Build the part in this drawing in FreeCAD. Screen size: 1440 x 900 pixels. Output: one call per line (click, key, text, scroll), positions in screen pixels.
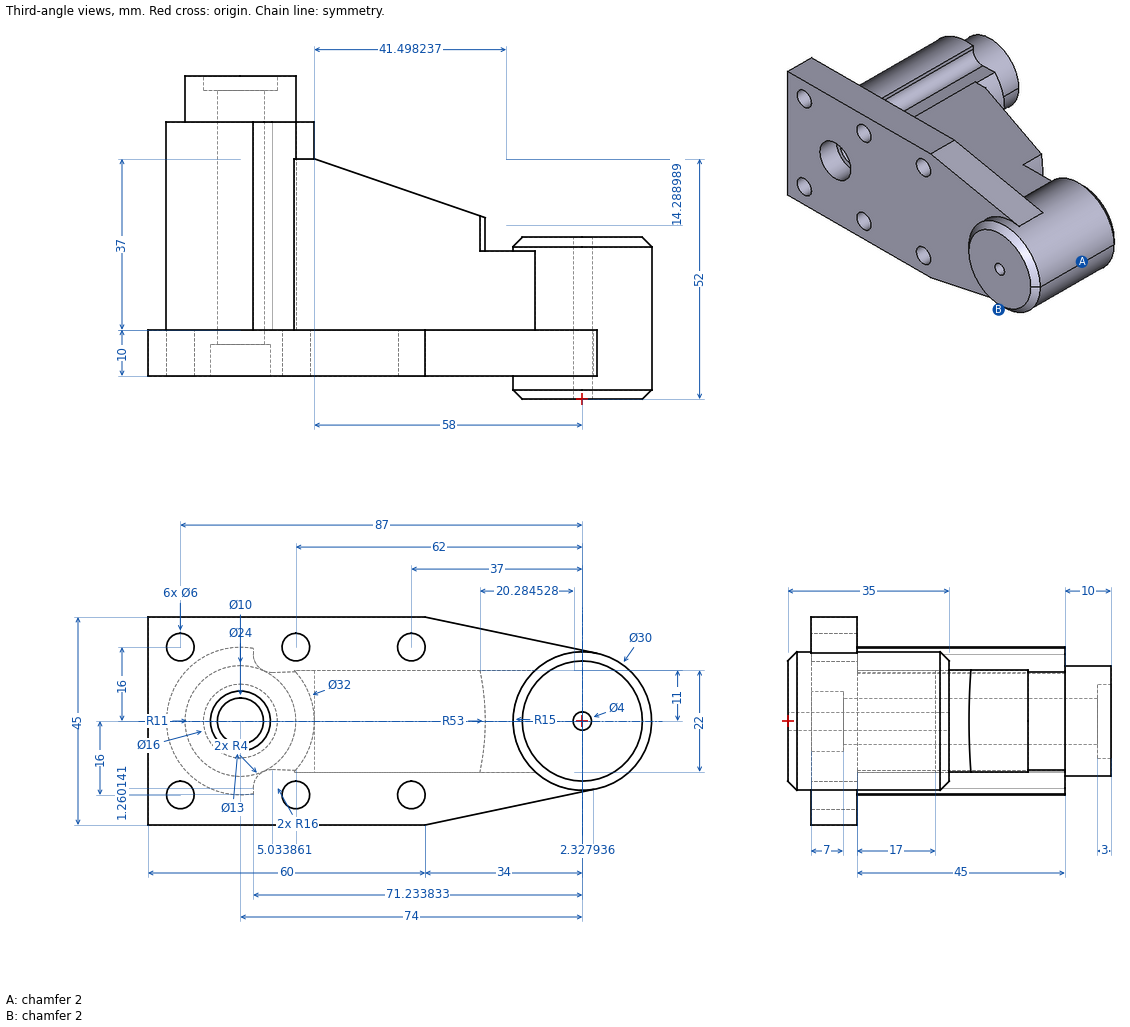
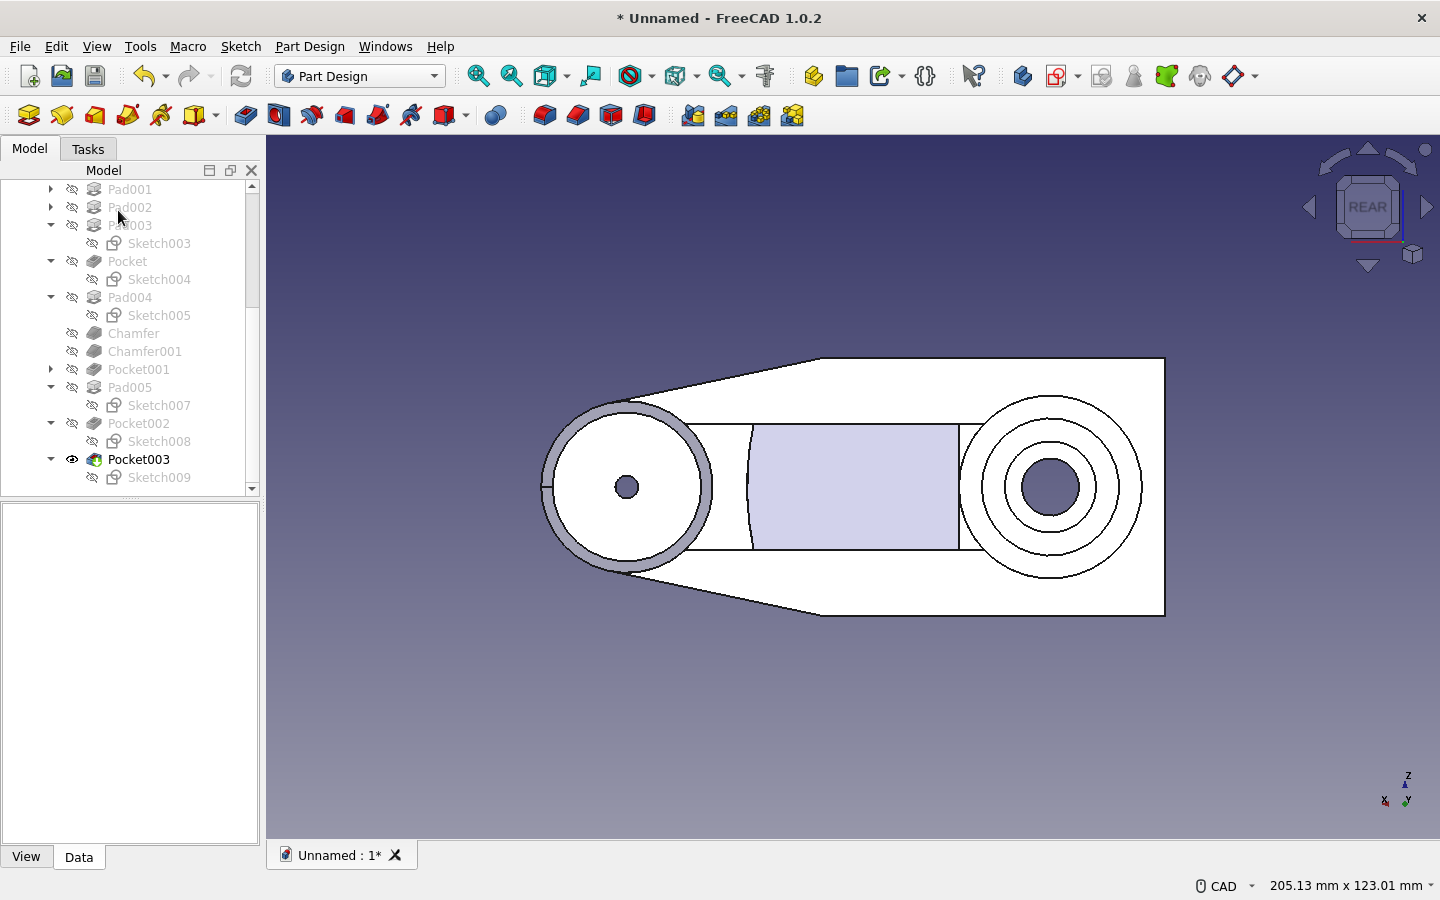
key(0)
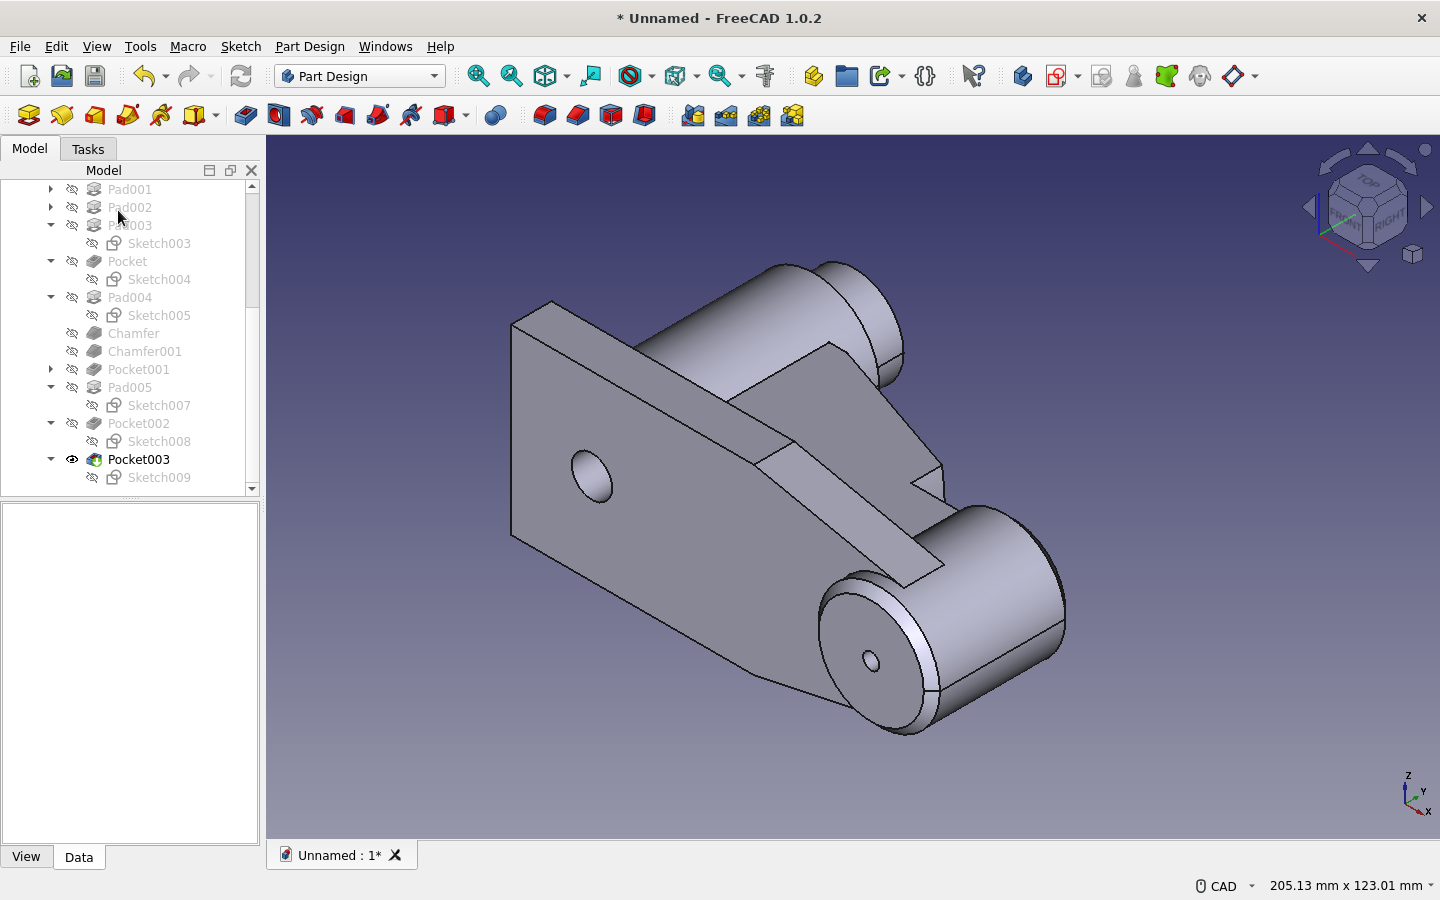
click(708, 542)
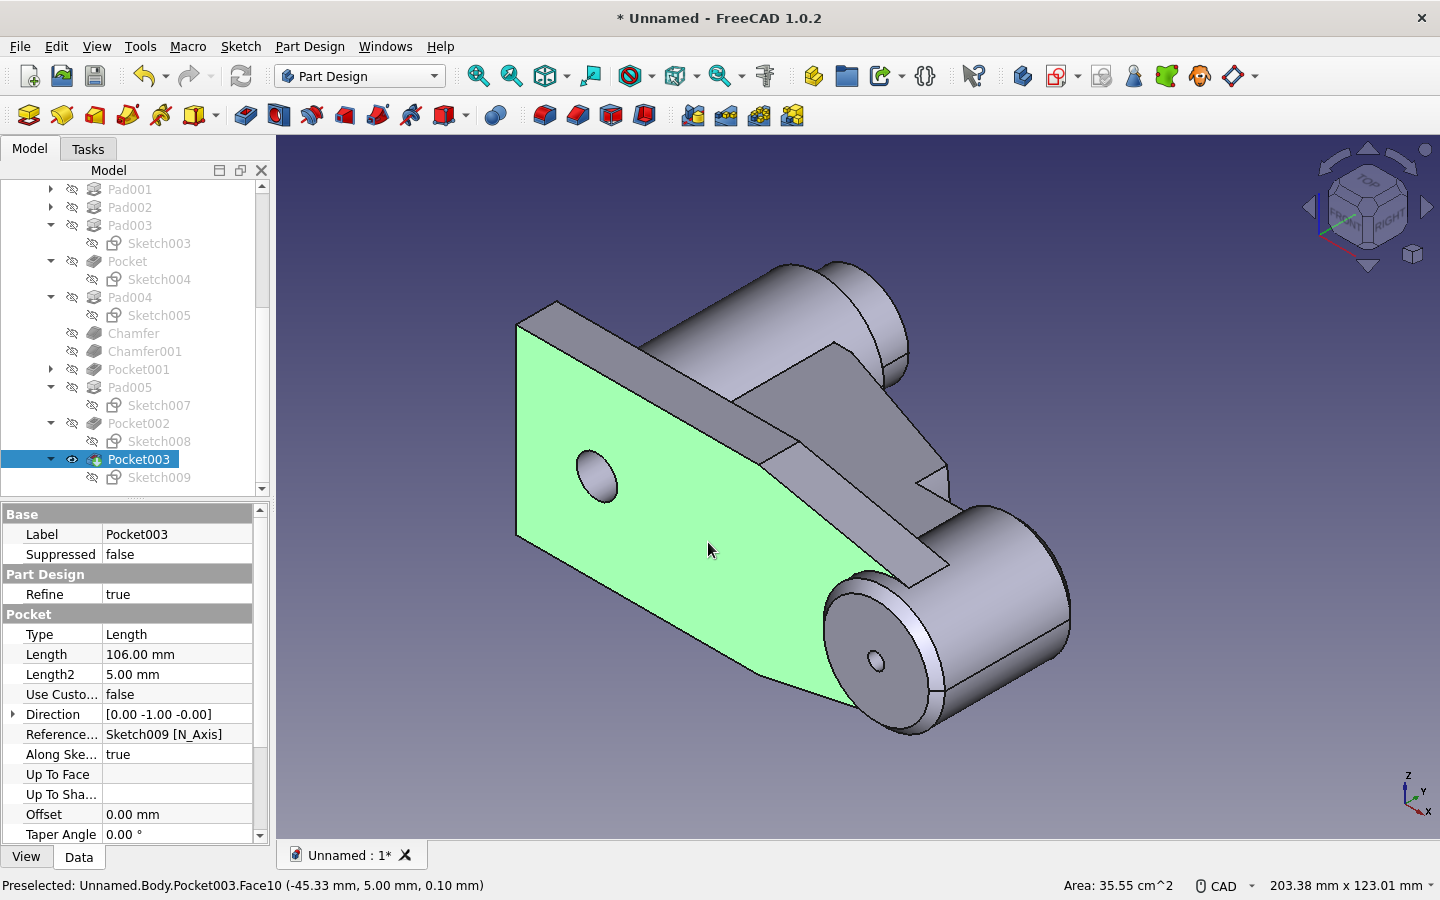
click(1056, 76)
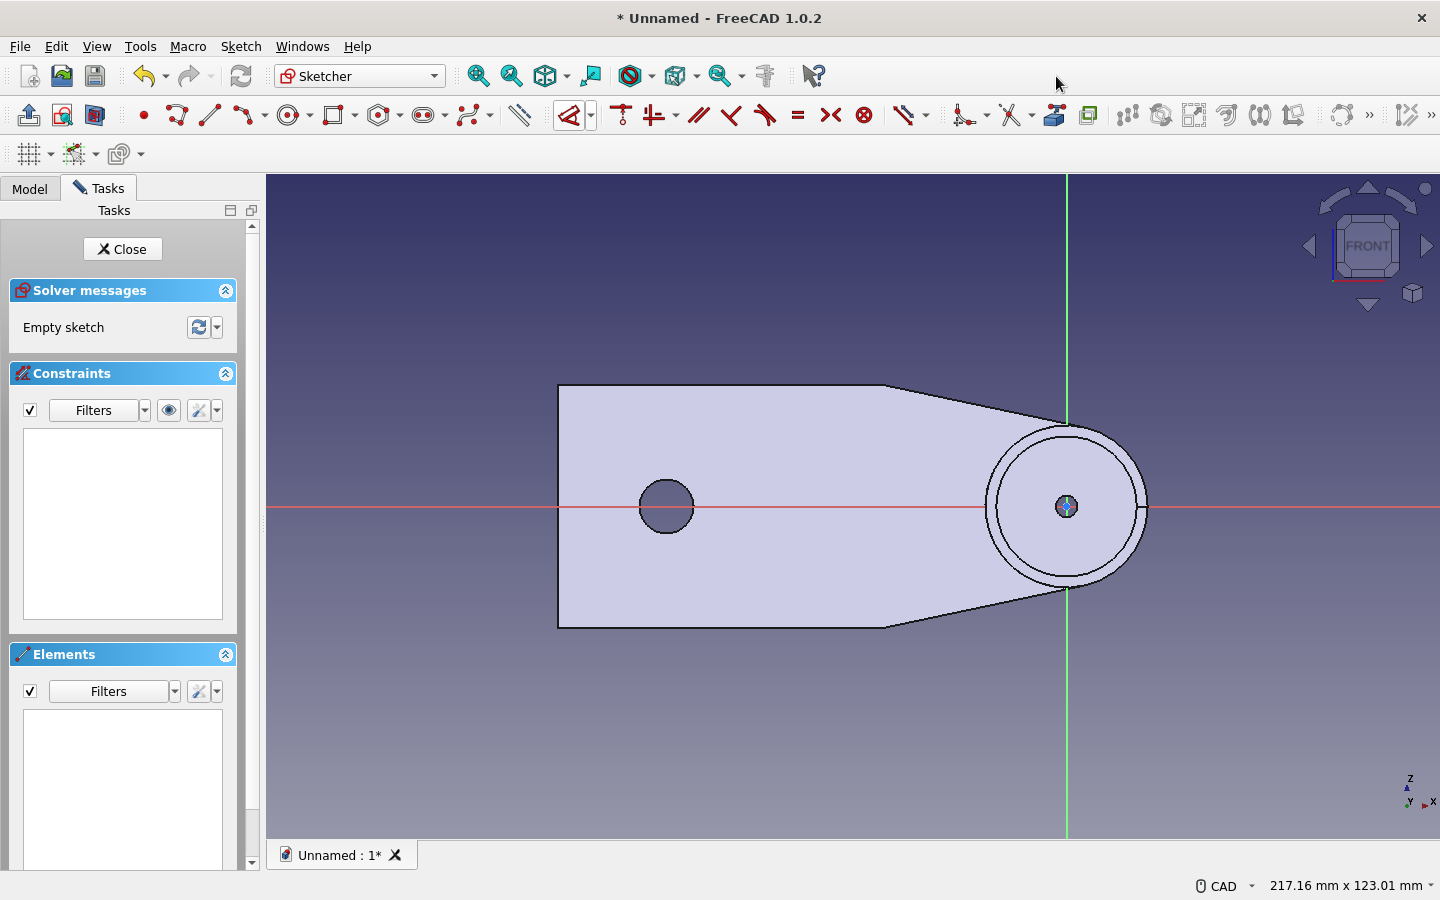
scroll(643, 507, up, 9)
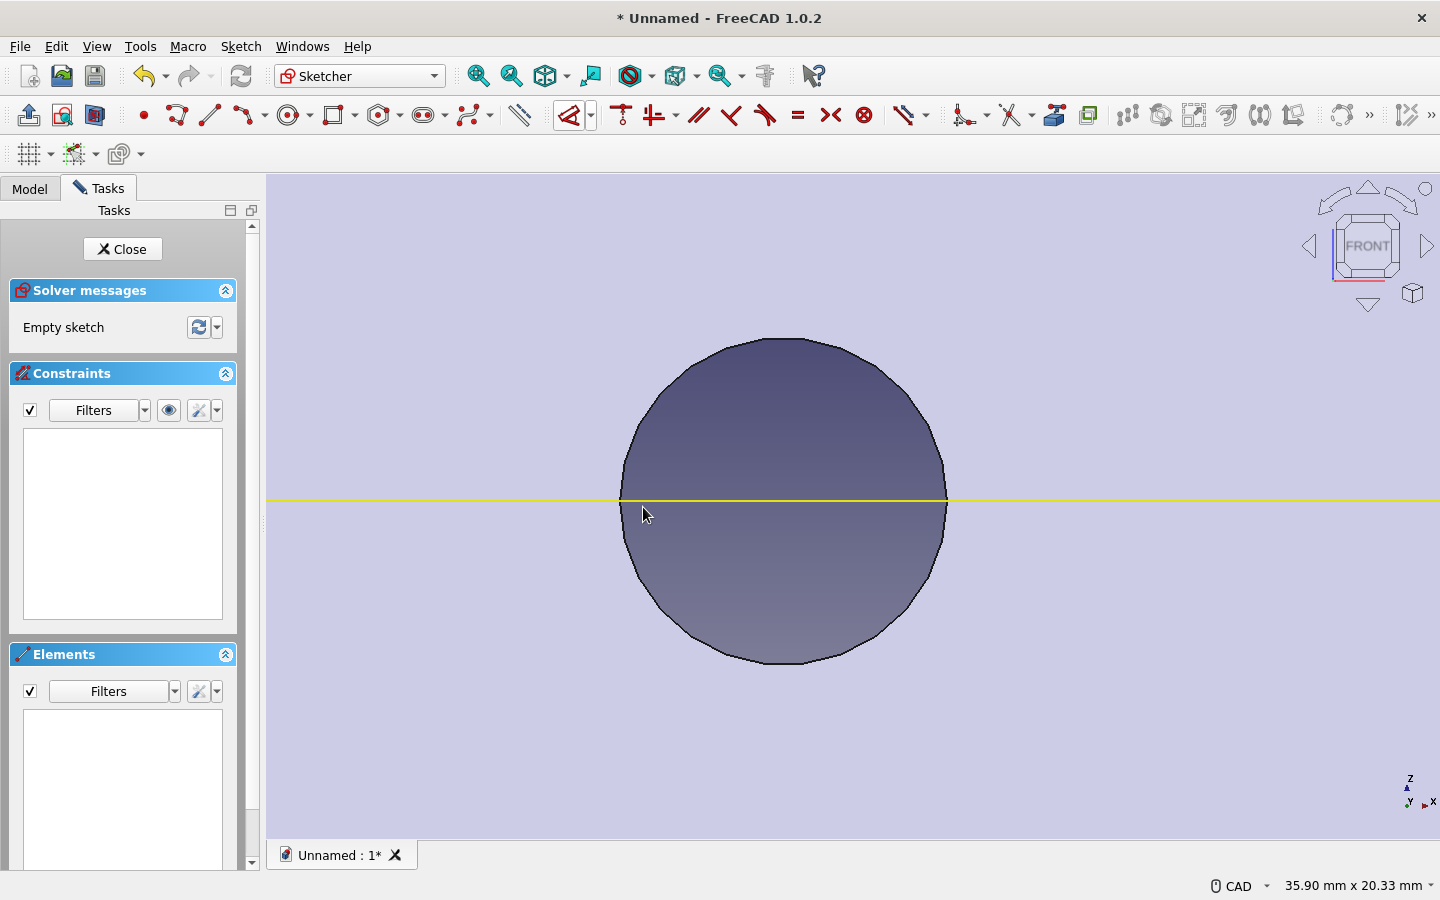
click(288, 116)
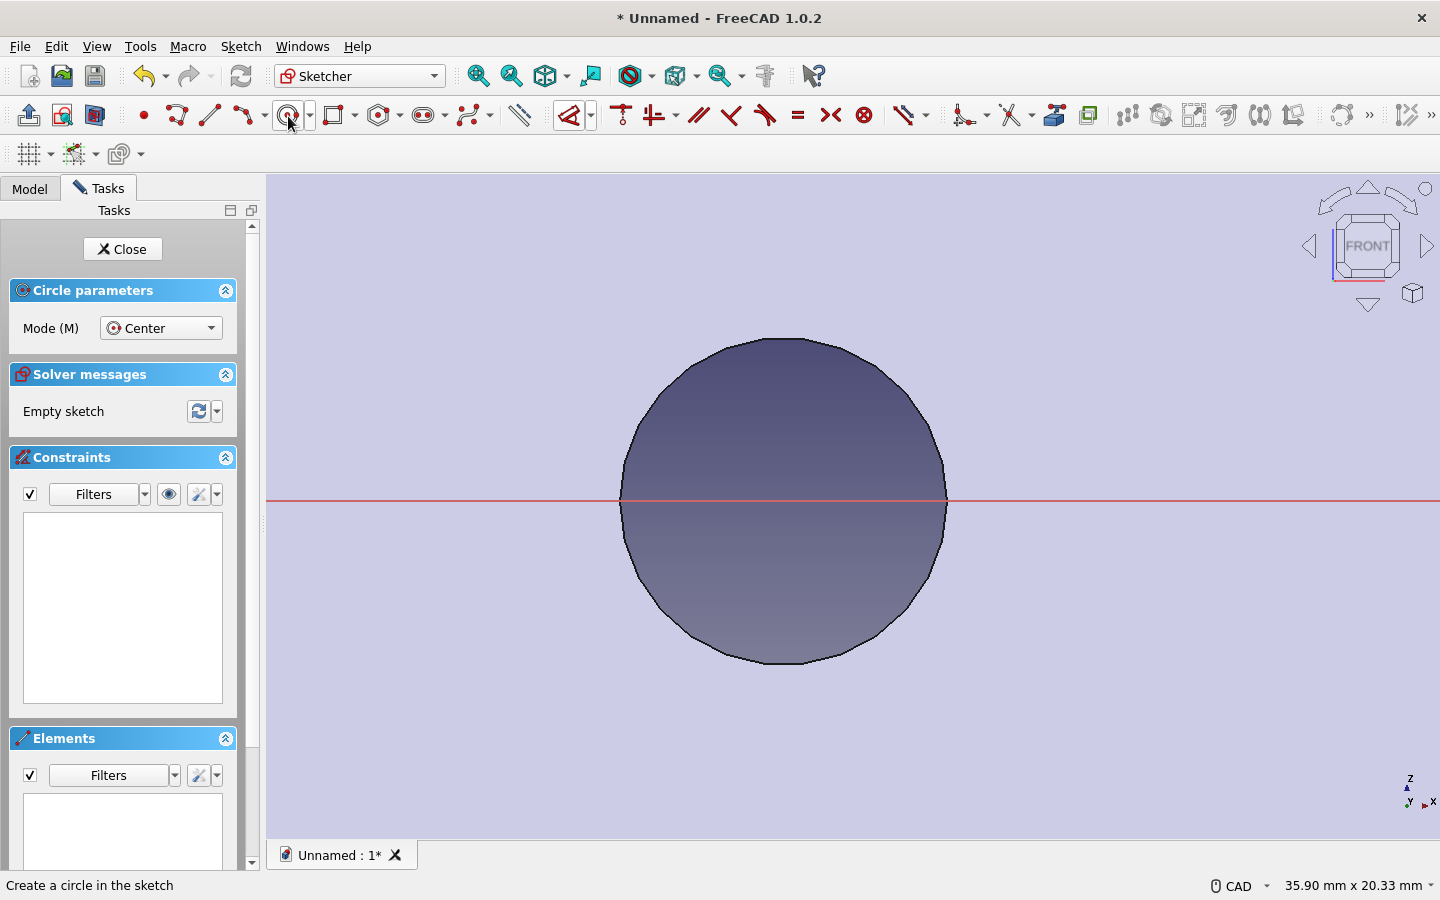
click(783, 501)
click(934, 351)
key(Escape)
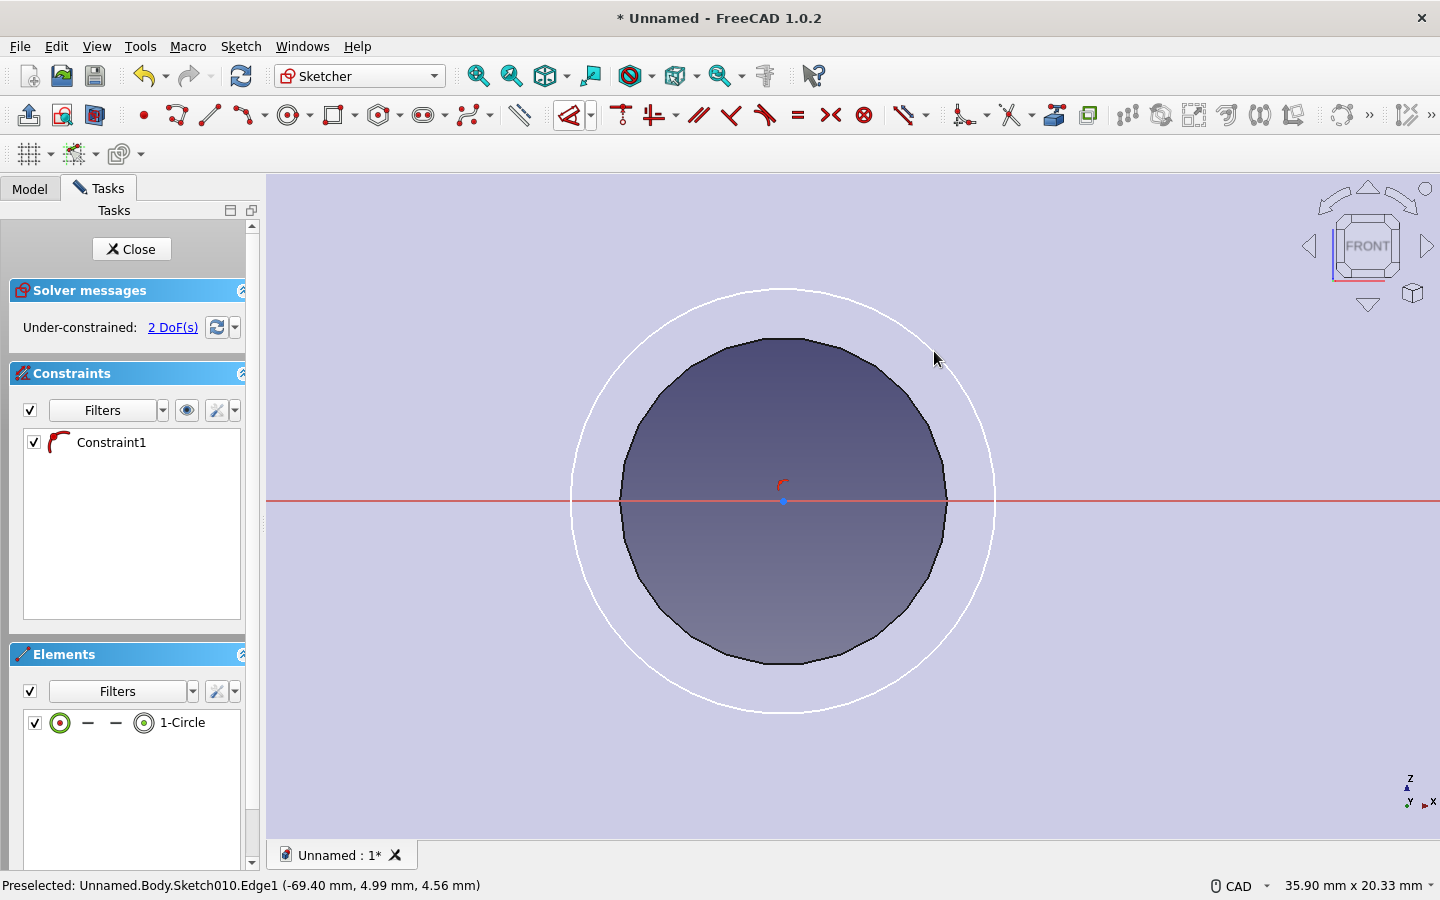
click(933, 351)